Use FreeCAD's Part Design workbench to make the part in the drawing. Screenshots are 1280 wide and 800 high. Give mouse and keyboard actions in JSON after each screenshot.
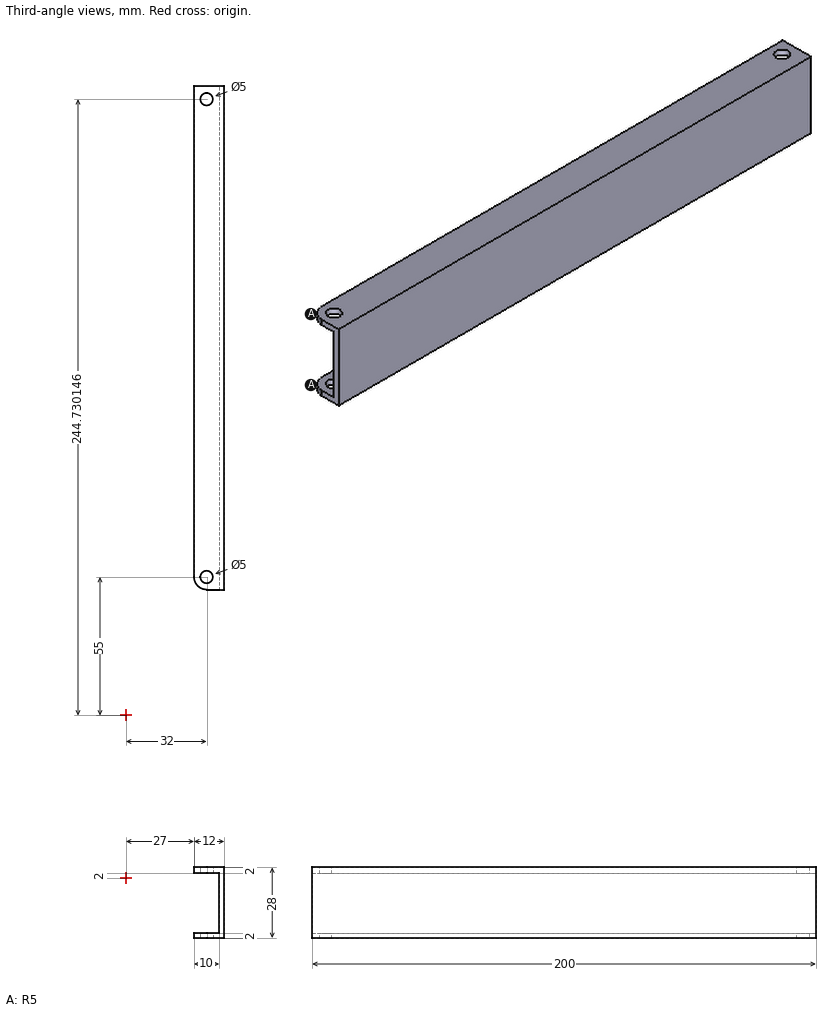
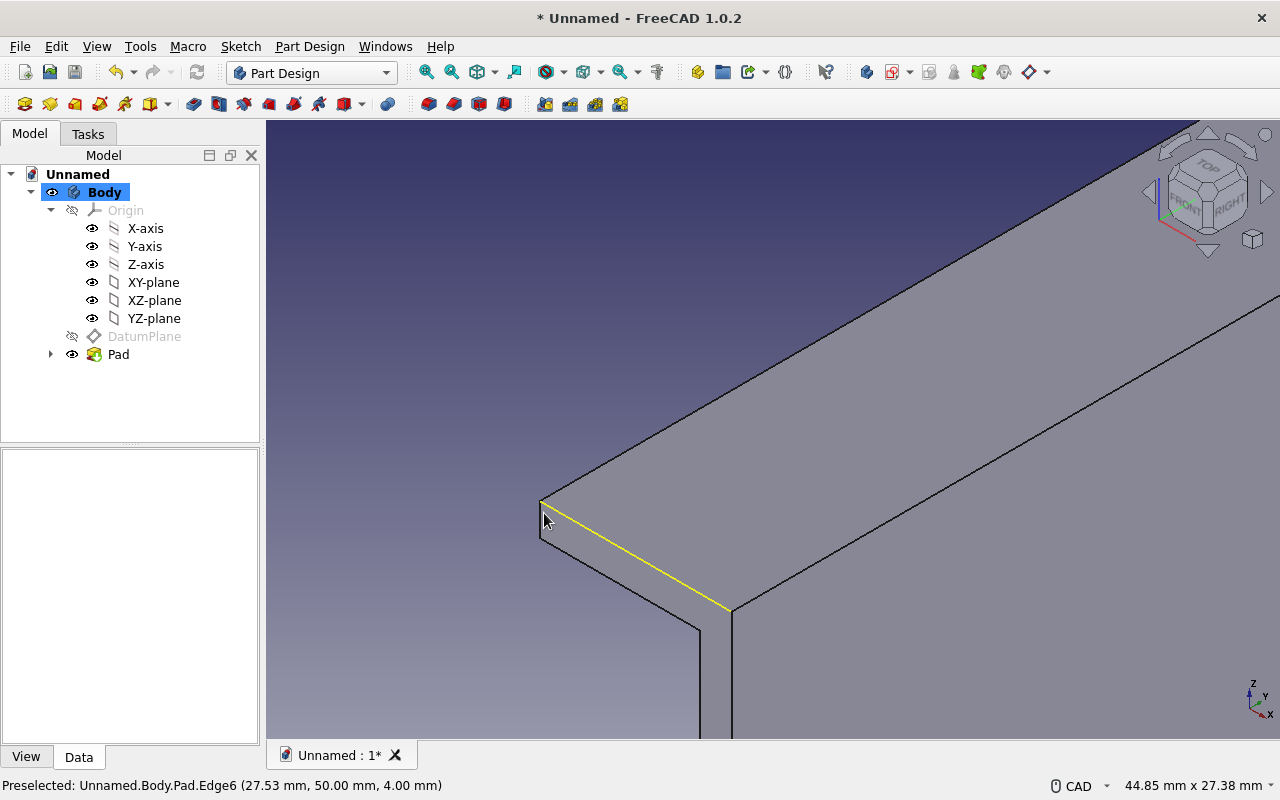
{"action": "left_click", "coordinate": [427, 72]}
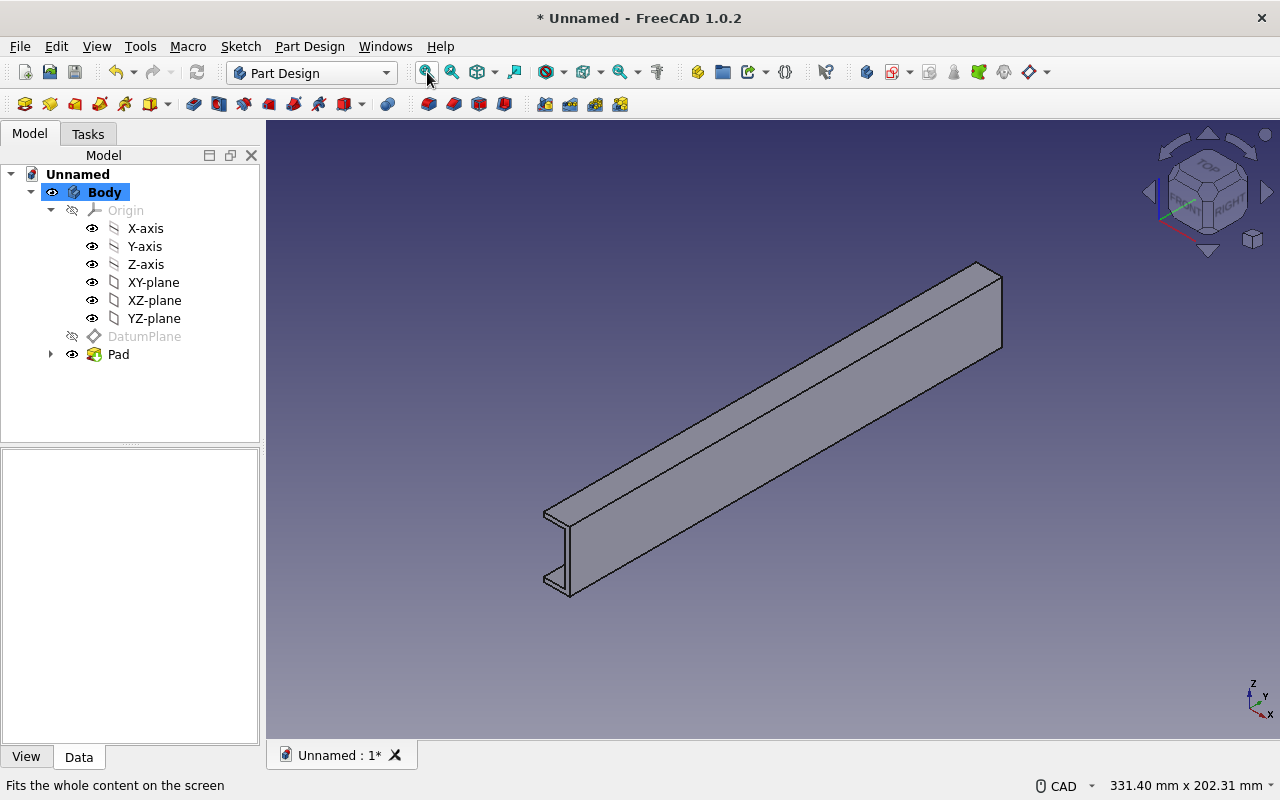
{"action": "key", "text": "2"}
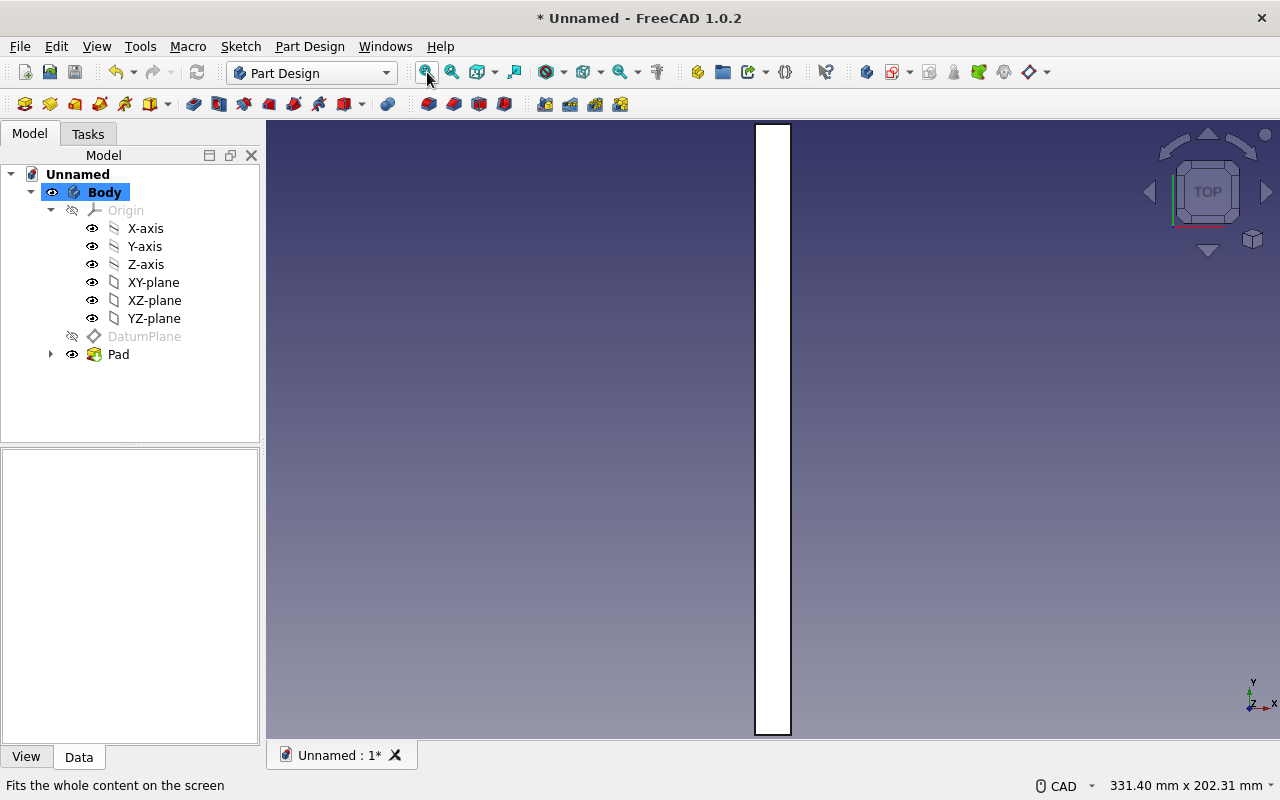
{"action": "key", "text": "1"}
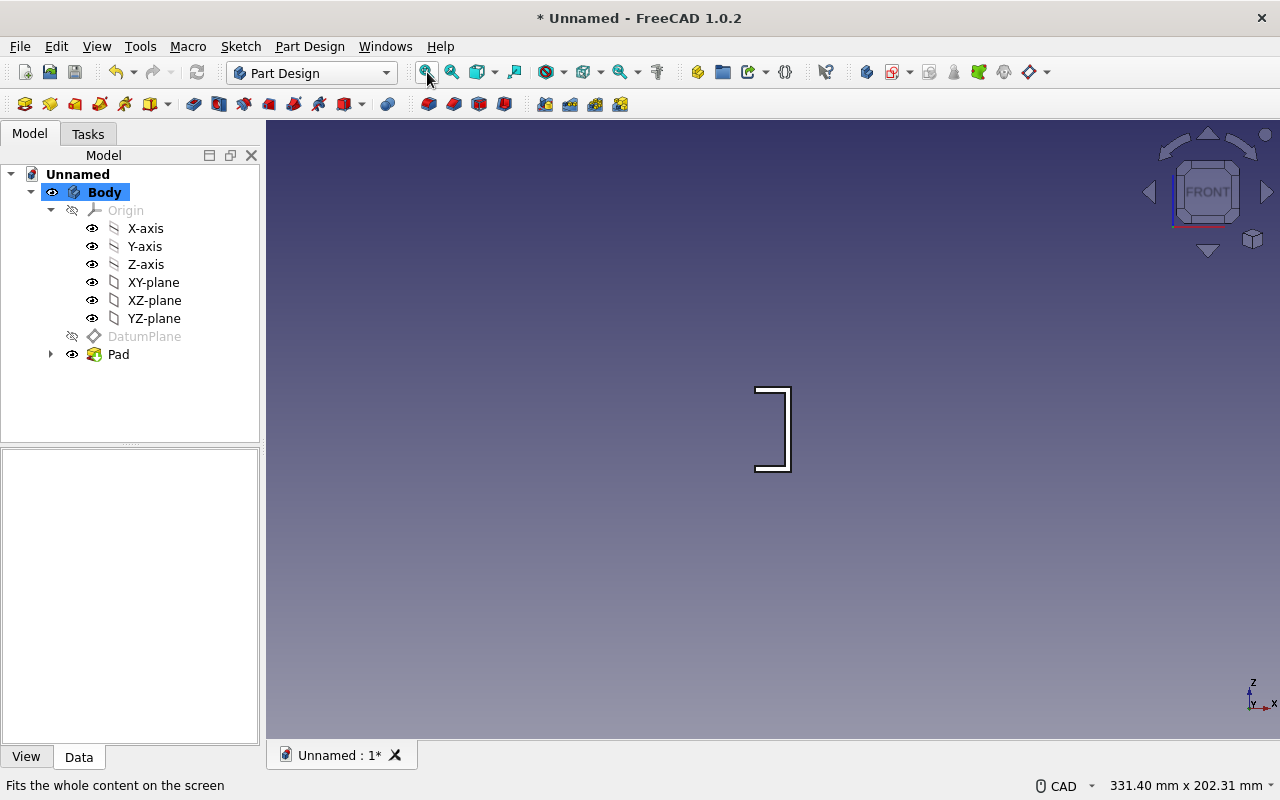
{"action": "left_click", "coordinate": [427, 72]}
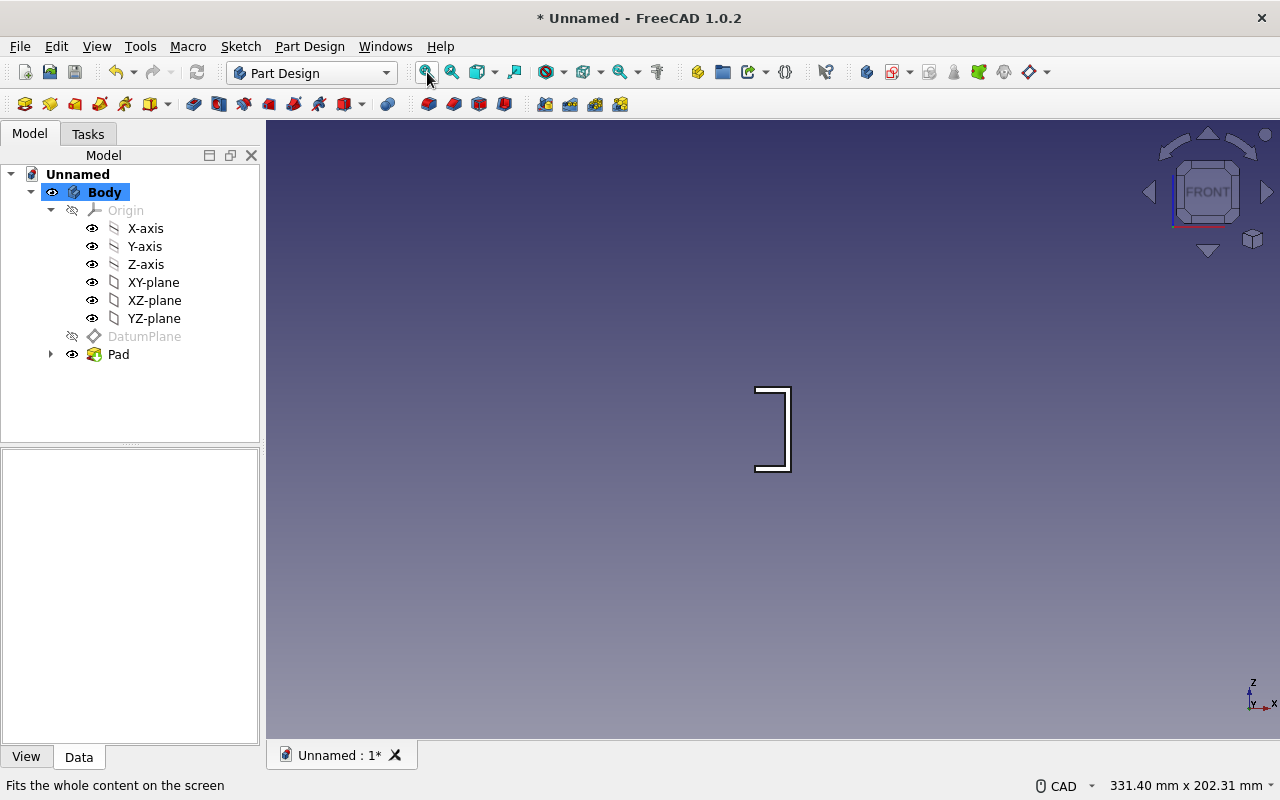
{"action": "scroll", "coordinate": [755, 389], "scroll_direction": "up", "scroll_amount": 10}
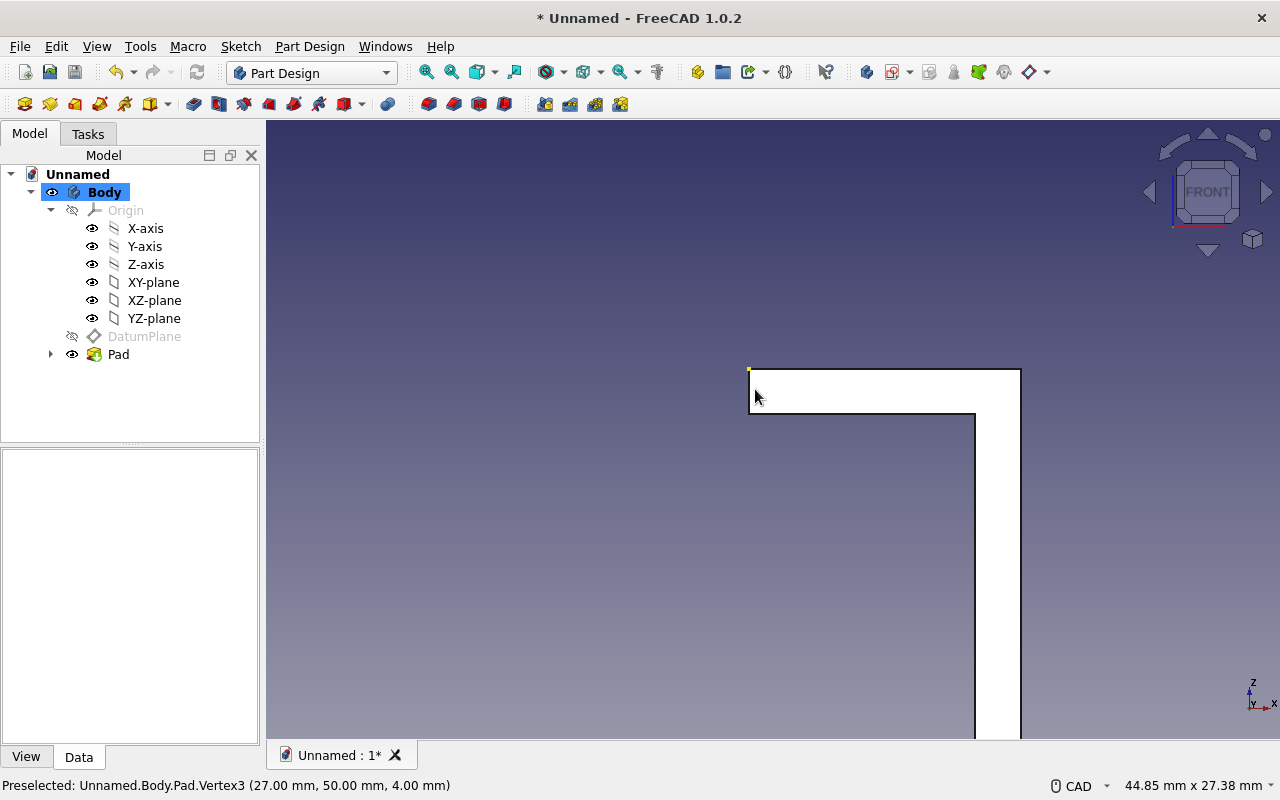
{"action": "left_click", "coordinate": [749, 391]}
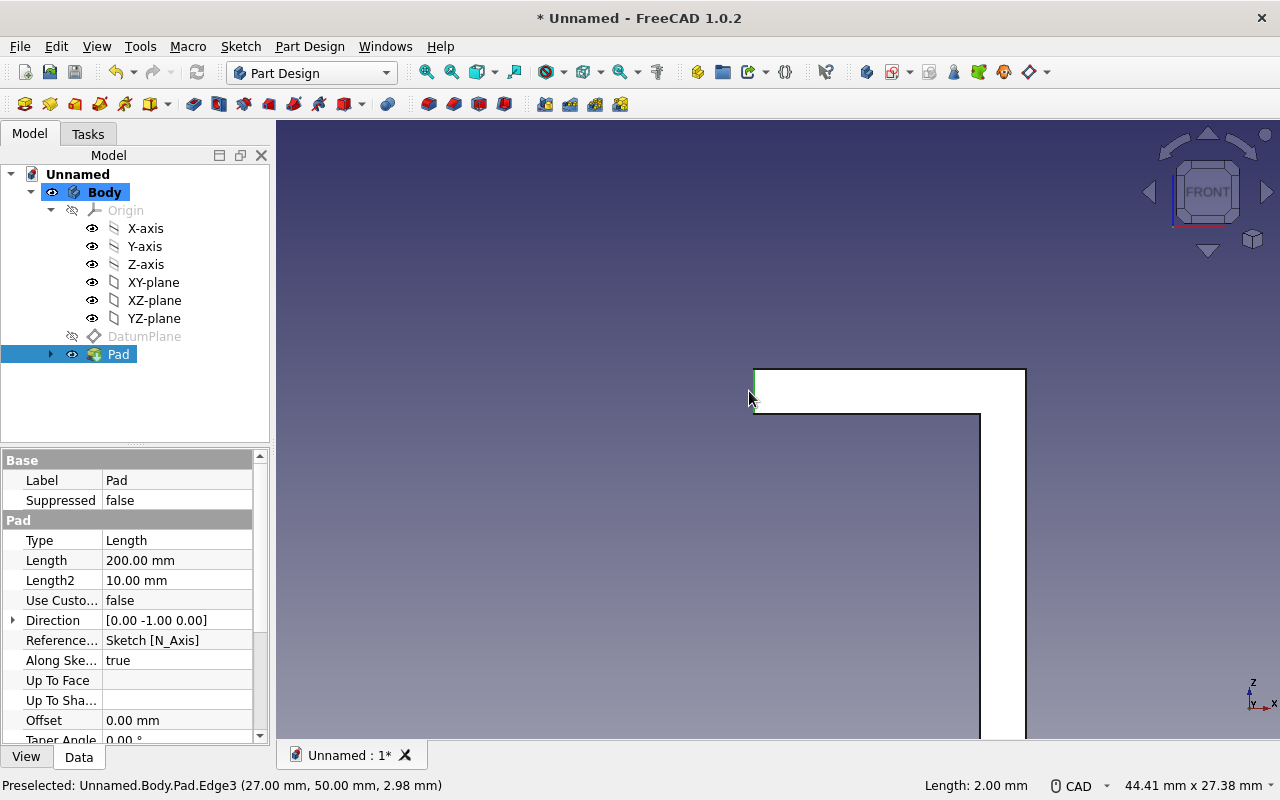
{"action": "left_click", "coordinate": [427, 72]}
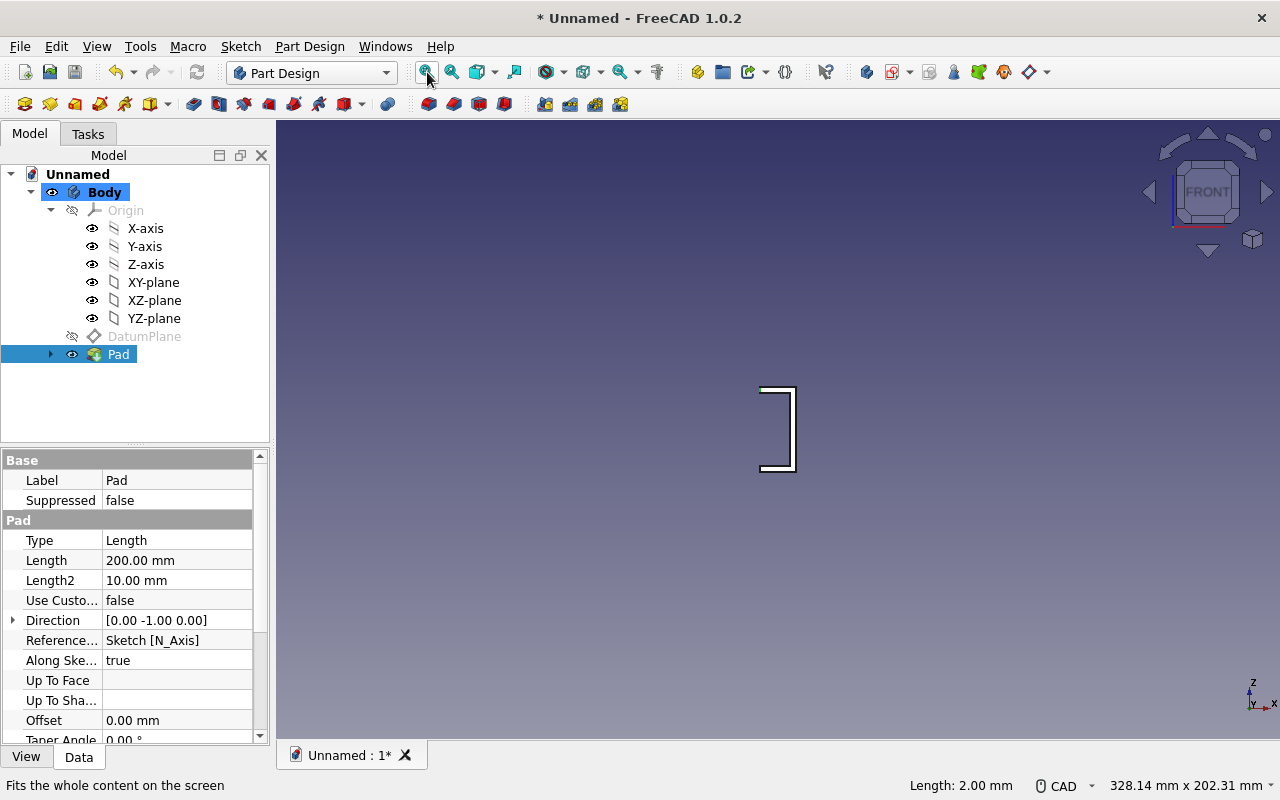
{"action": "key", "text": "3"}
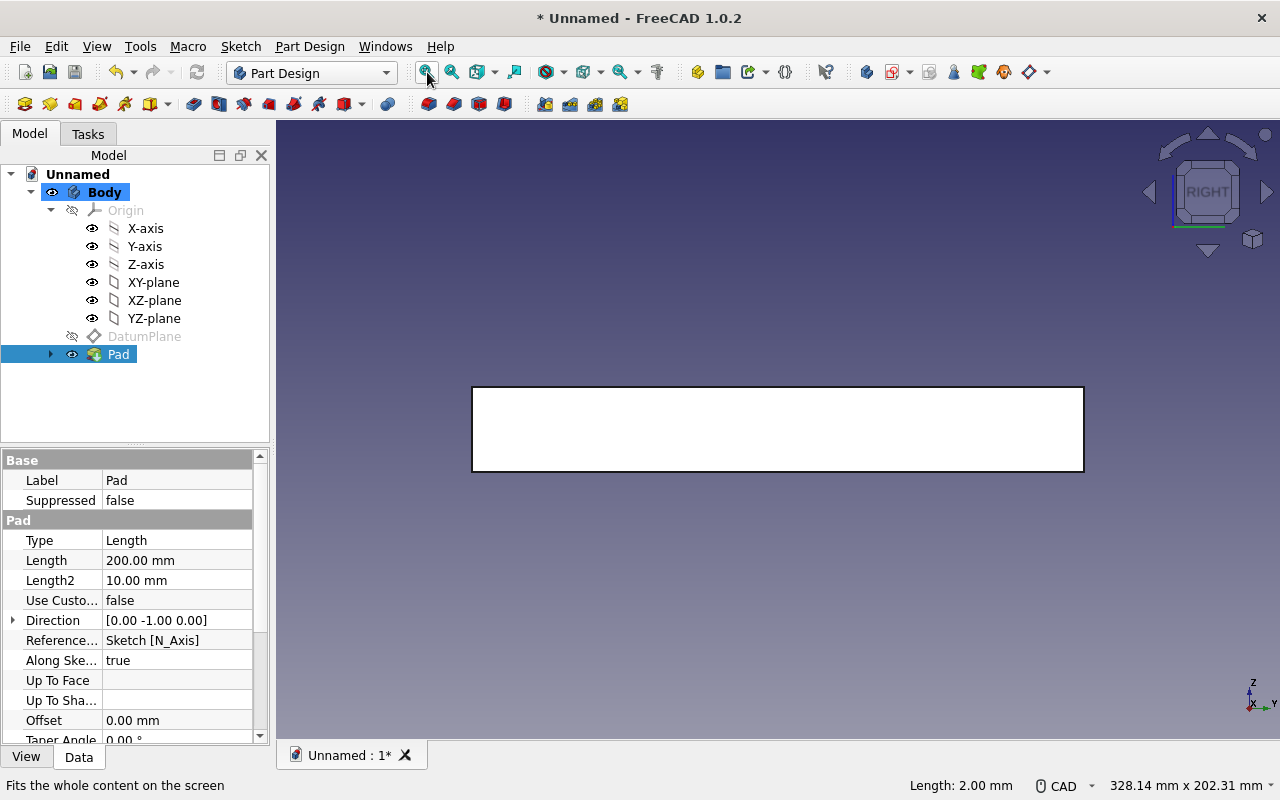
{"action": "scroll", "coordinate": [472, 468], "scroll_direction": "up", "scroll_amount": 10}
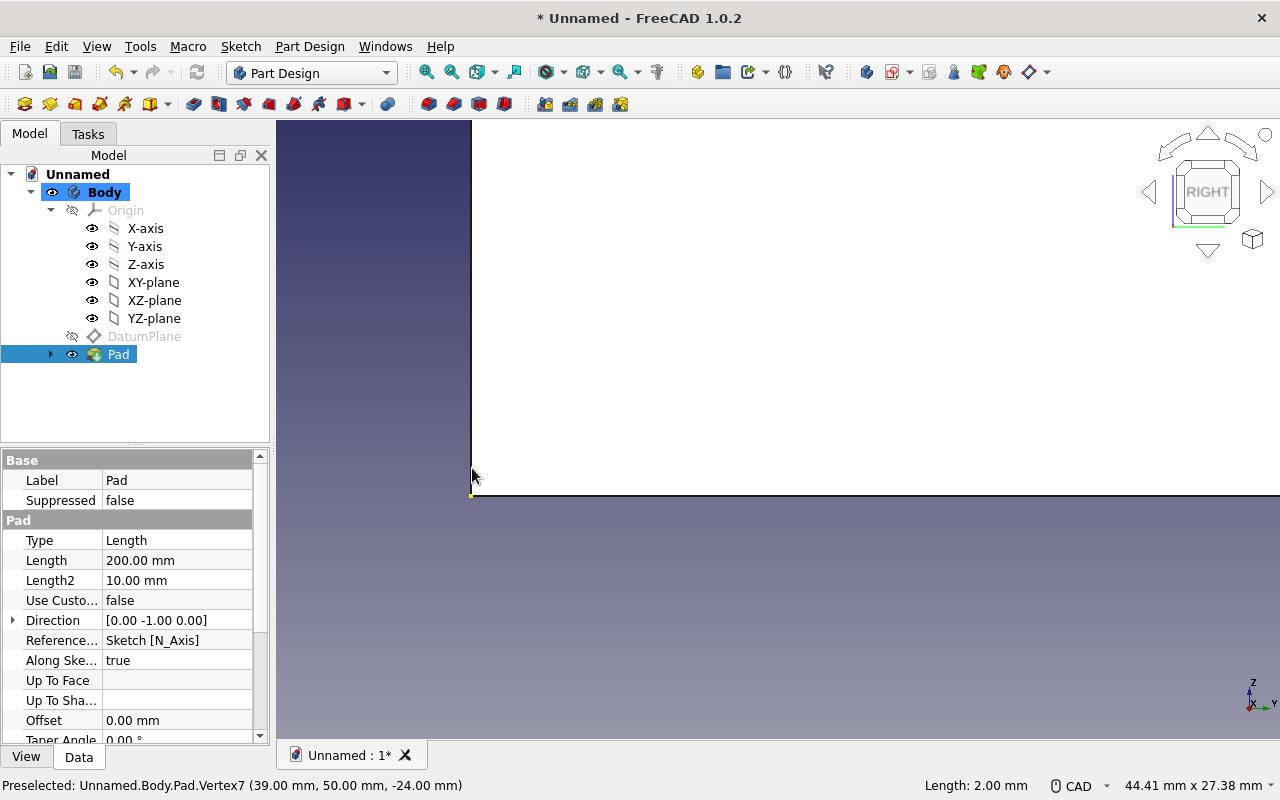
{"action": "left_click", "coordinate": [427, 72]}